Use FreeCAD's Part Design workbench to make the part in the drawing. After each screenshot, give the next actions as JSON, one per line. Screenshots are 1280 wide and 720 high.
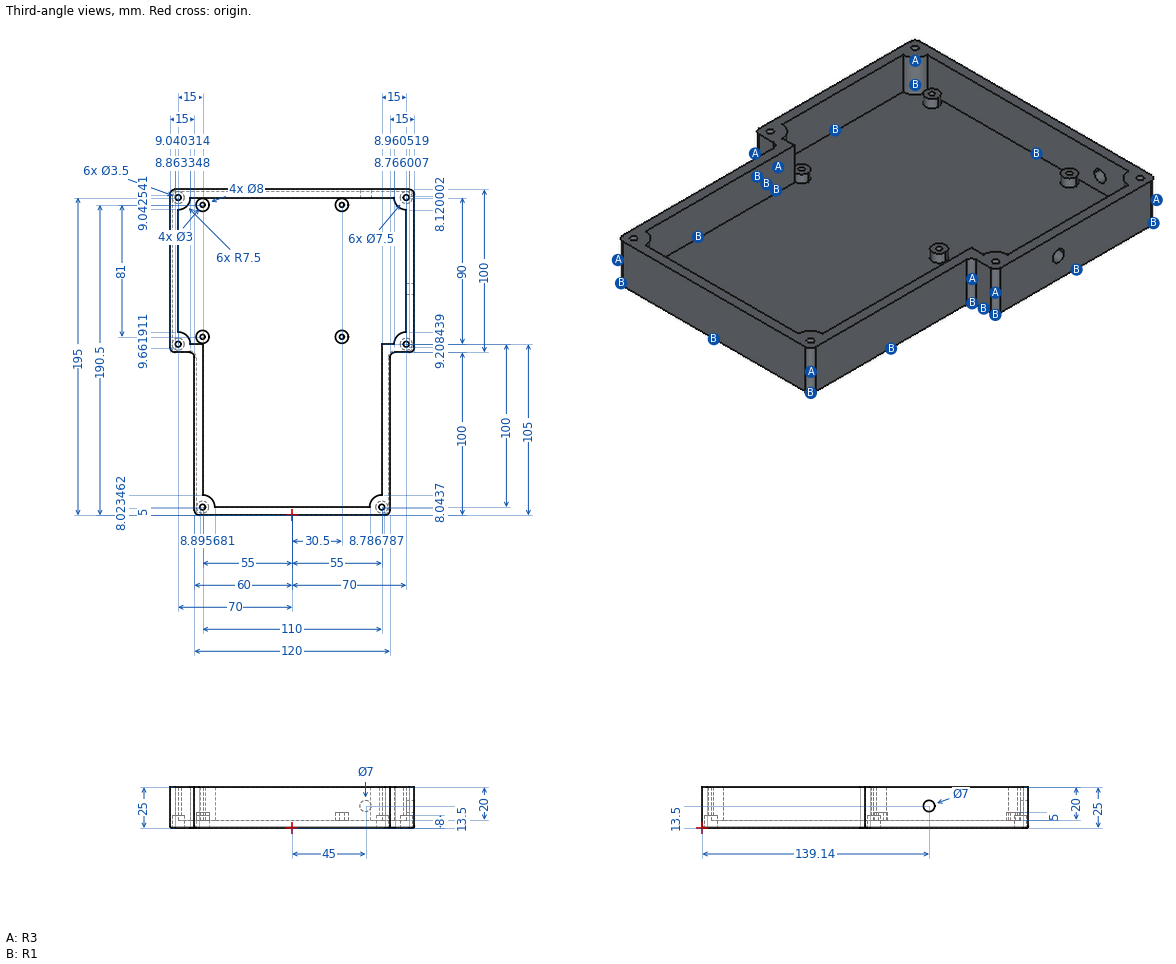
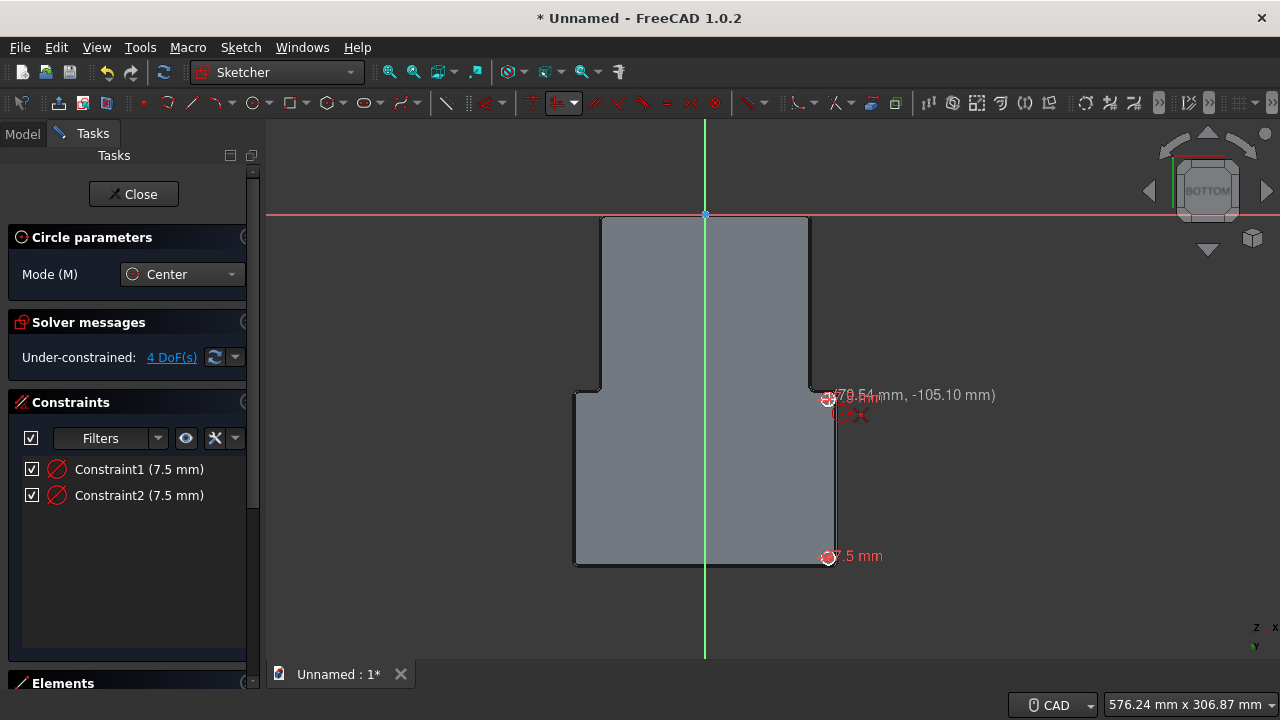
{"action": "scroll", "coordinate": [802, 223], "scroll_direction": "up", "scroll_amount": 7}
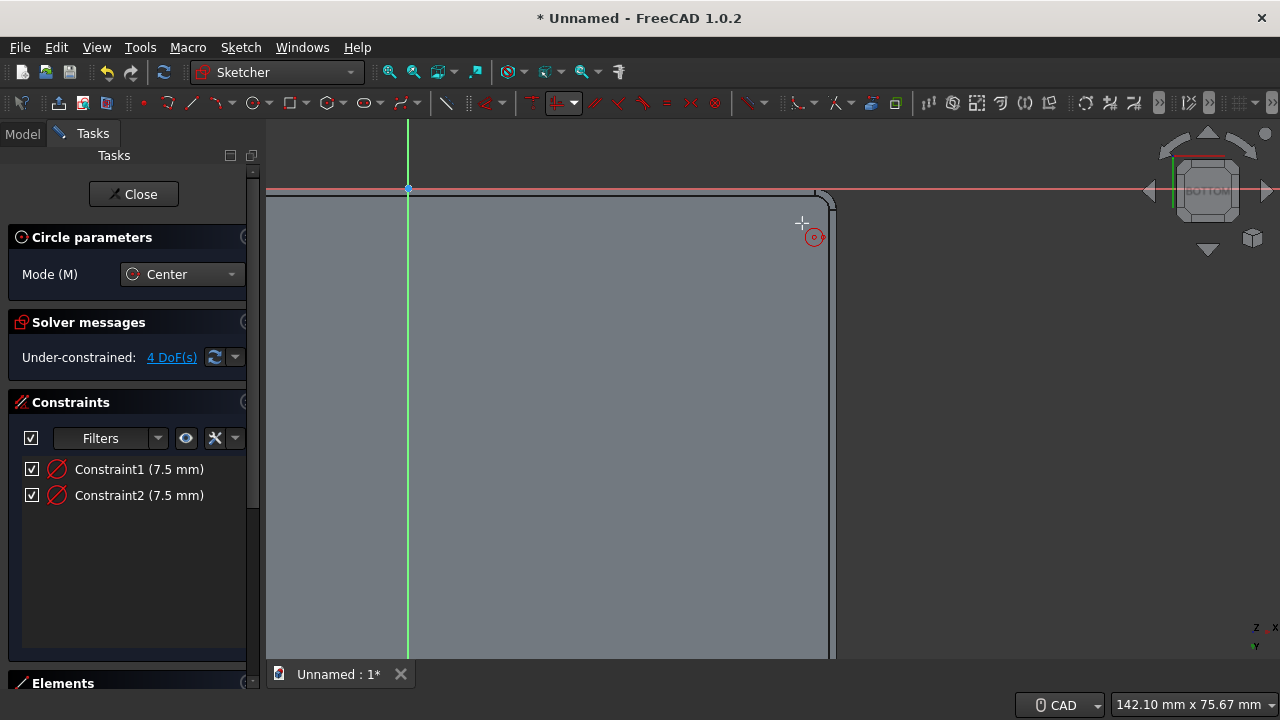
{"action": "left_click", "coordinate": [801, 224]}
{"action": "mouse_move", "coordinate": [820, 205]}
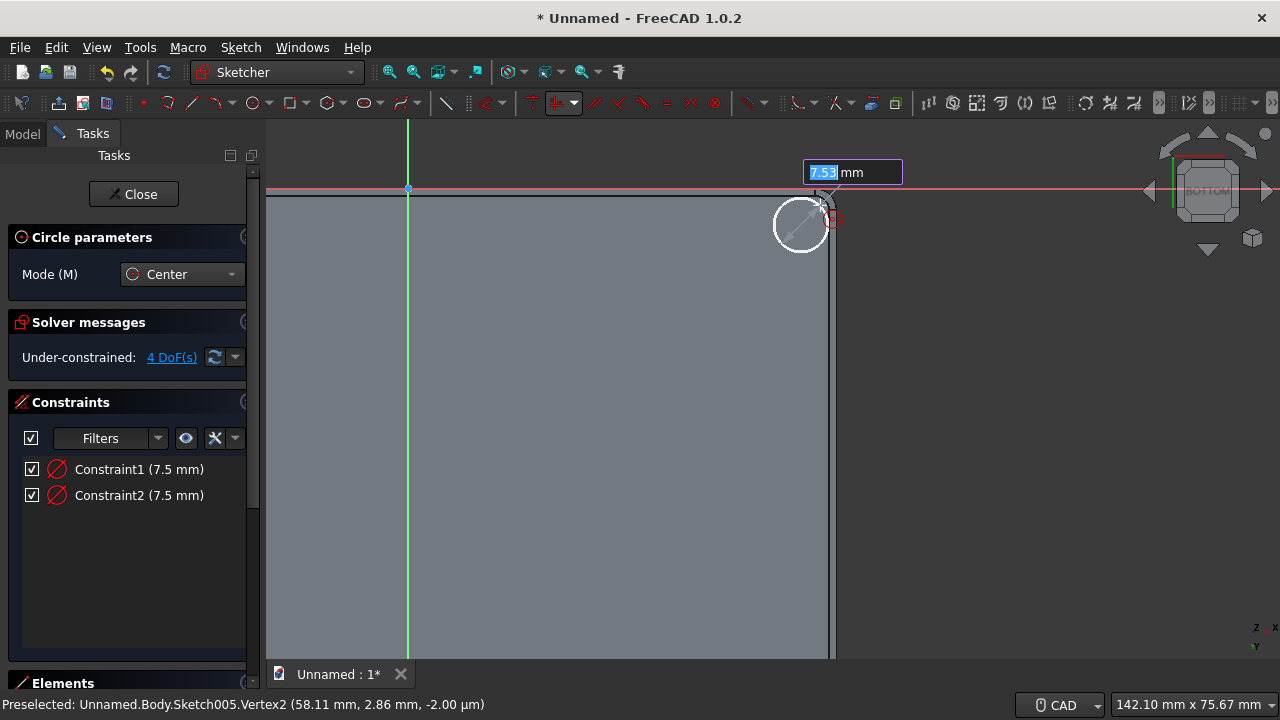
{"action": "type", "text": "7.5"}
{"action": "key", "text": "Return"}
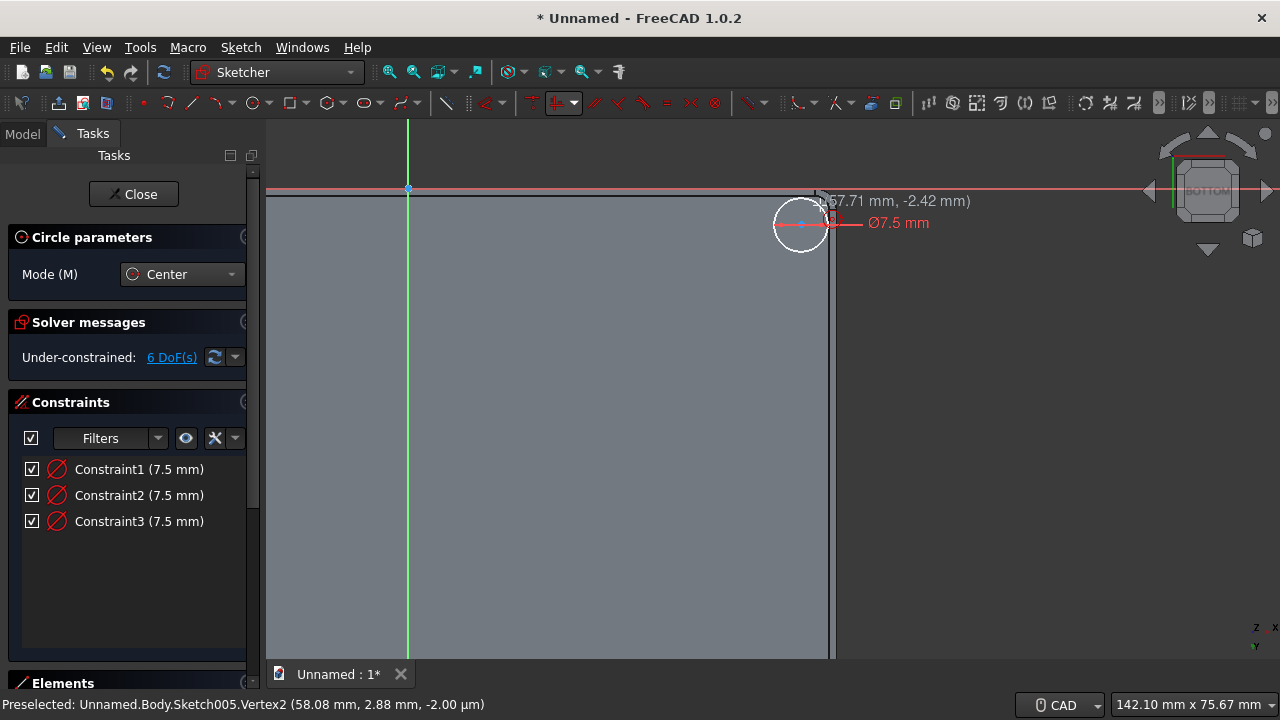
{"action": "scroll", "coordinate": [801, 222], "scroll_direction": "down", "scroll_amount": 7}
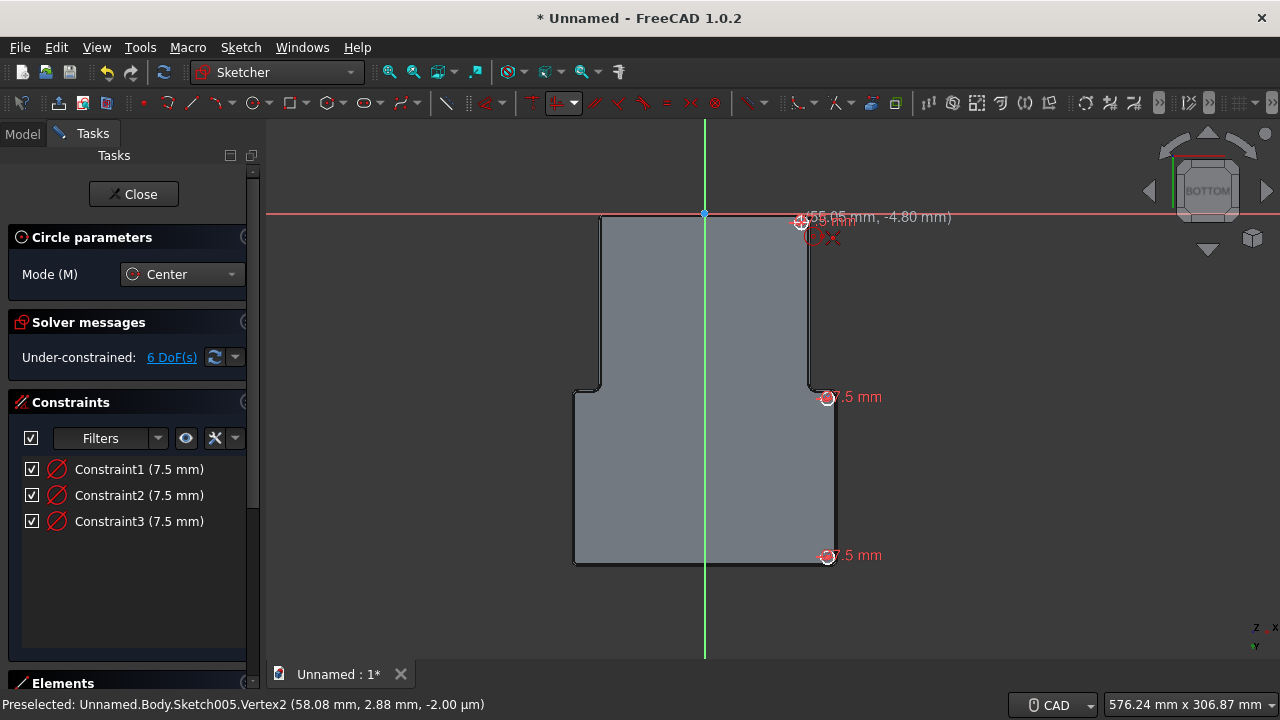
{"action": "scroll", "coordinate": [608, 223], "scroll_direction": "up", "scroll_amount": 7}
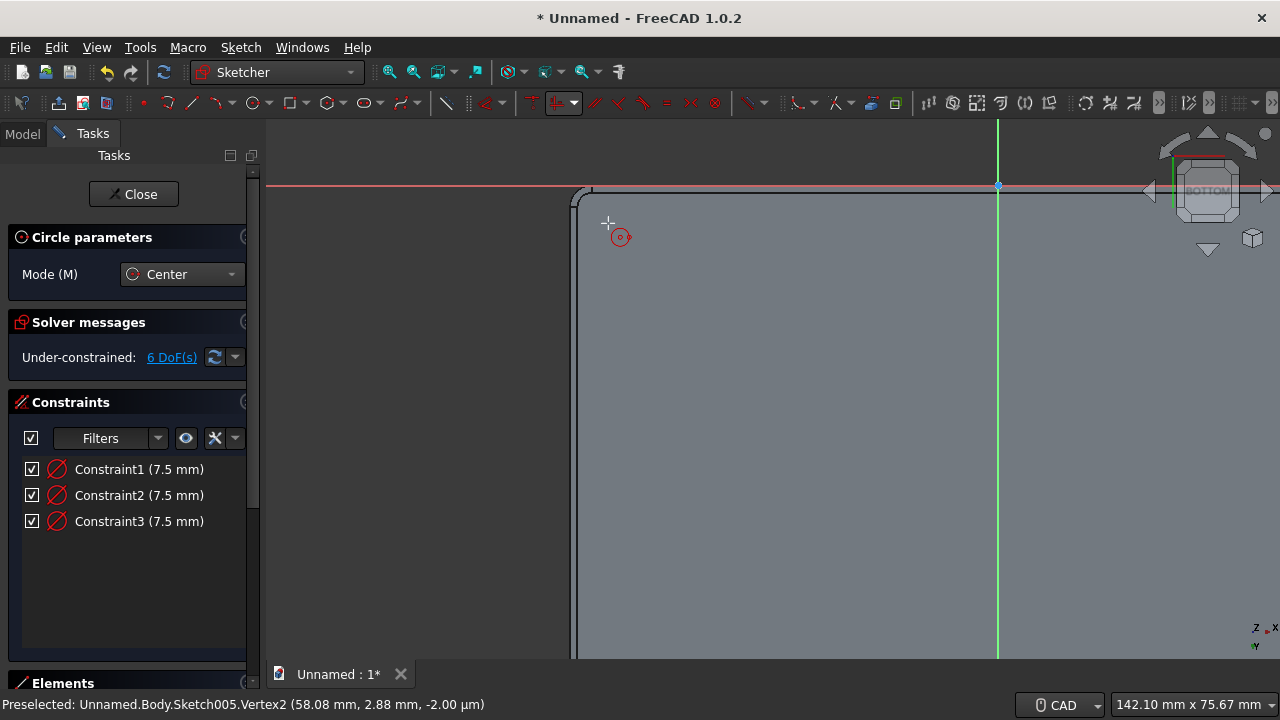
{"action": "left_click", "coordinate": [606, 221]}
{"action": "mouse_move", "coordinate": [625, 202]}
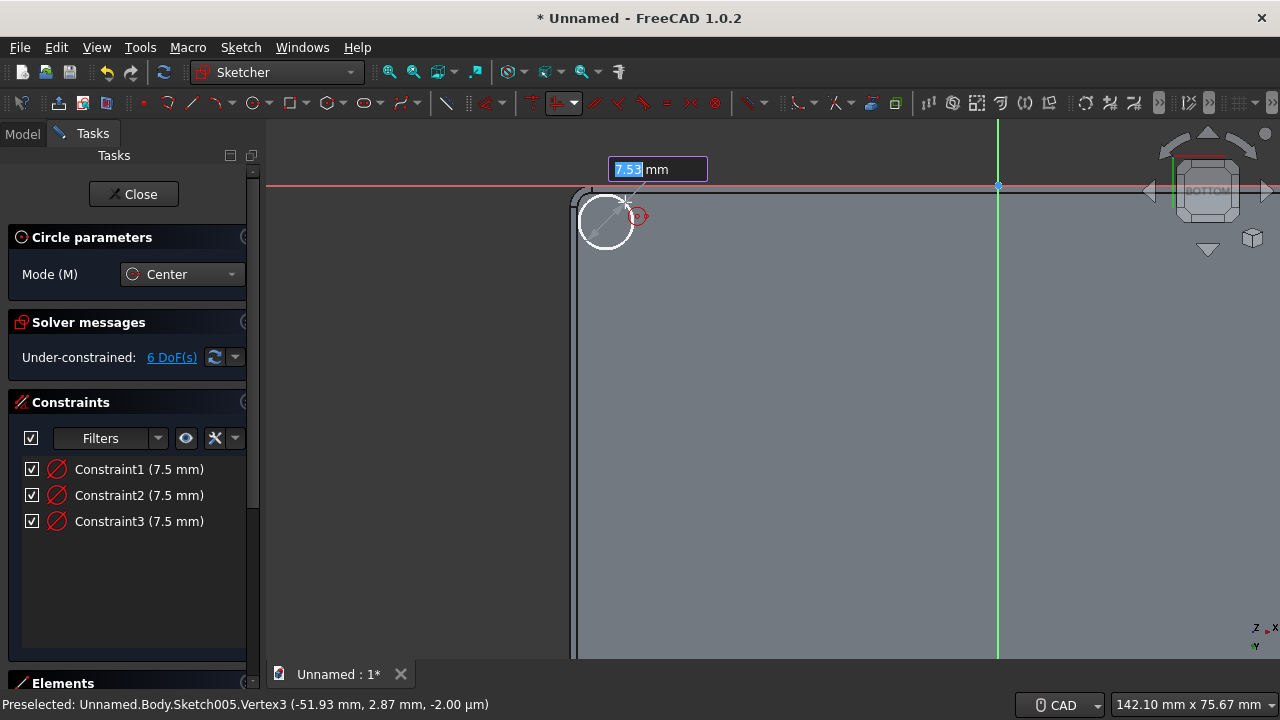
{"action": "type", "text": "7.5"}
{"action": "key", "text": "Return"}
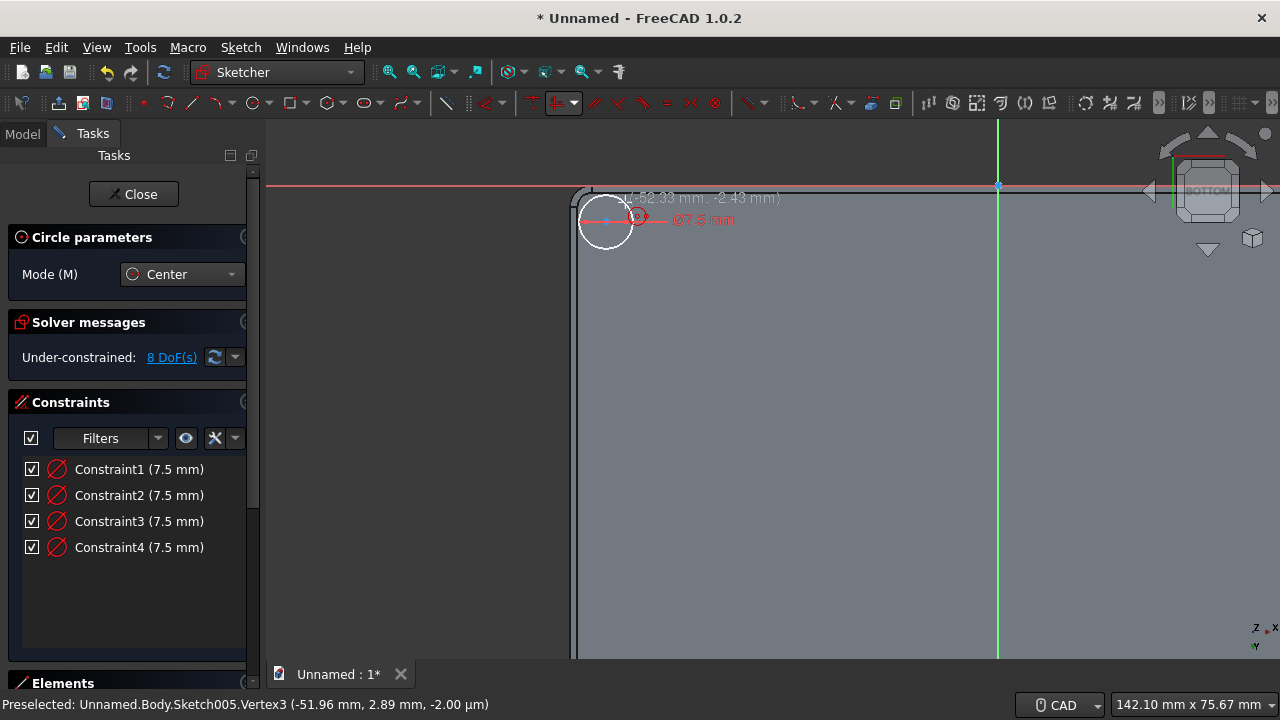
{"action": "scroll", "coordinate": [608, 223], "scroll_direction": "down", "scroll_amount": 7}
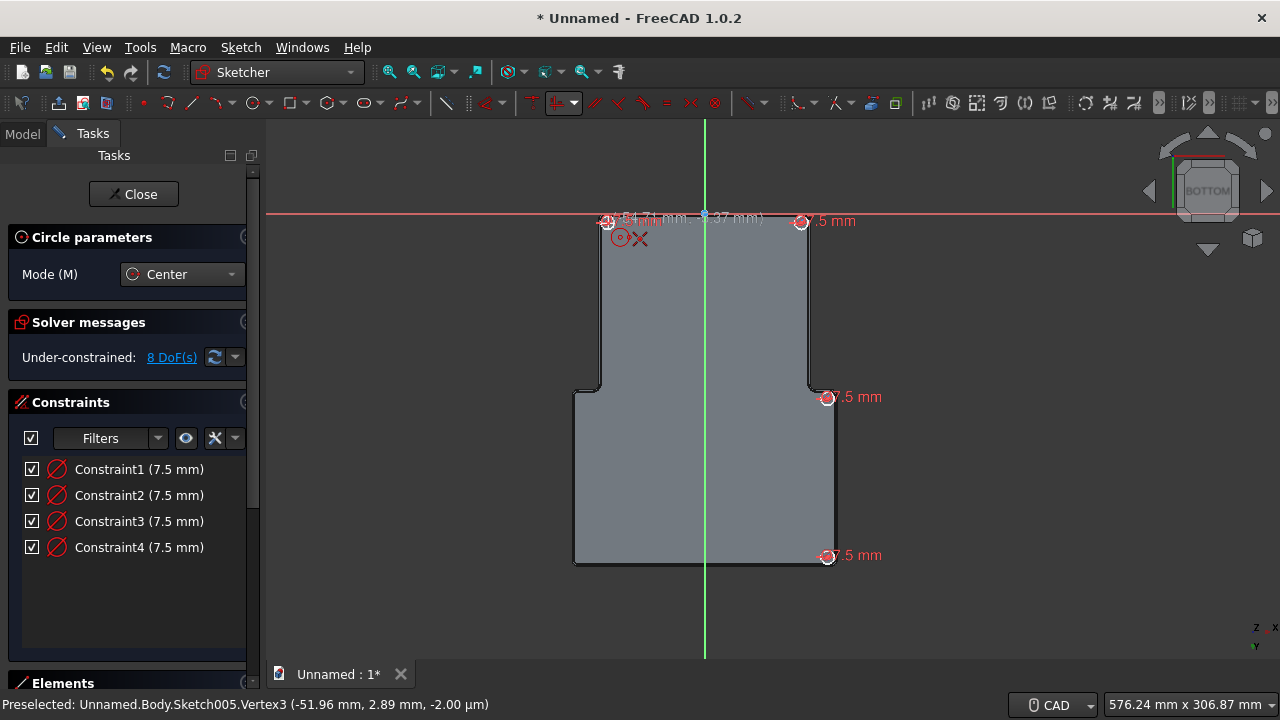
{"action": "scroll", "coordinate": [581, 399], "scroll_direction": "up", "scroll_amount": 7}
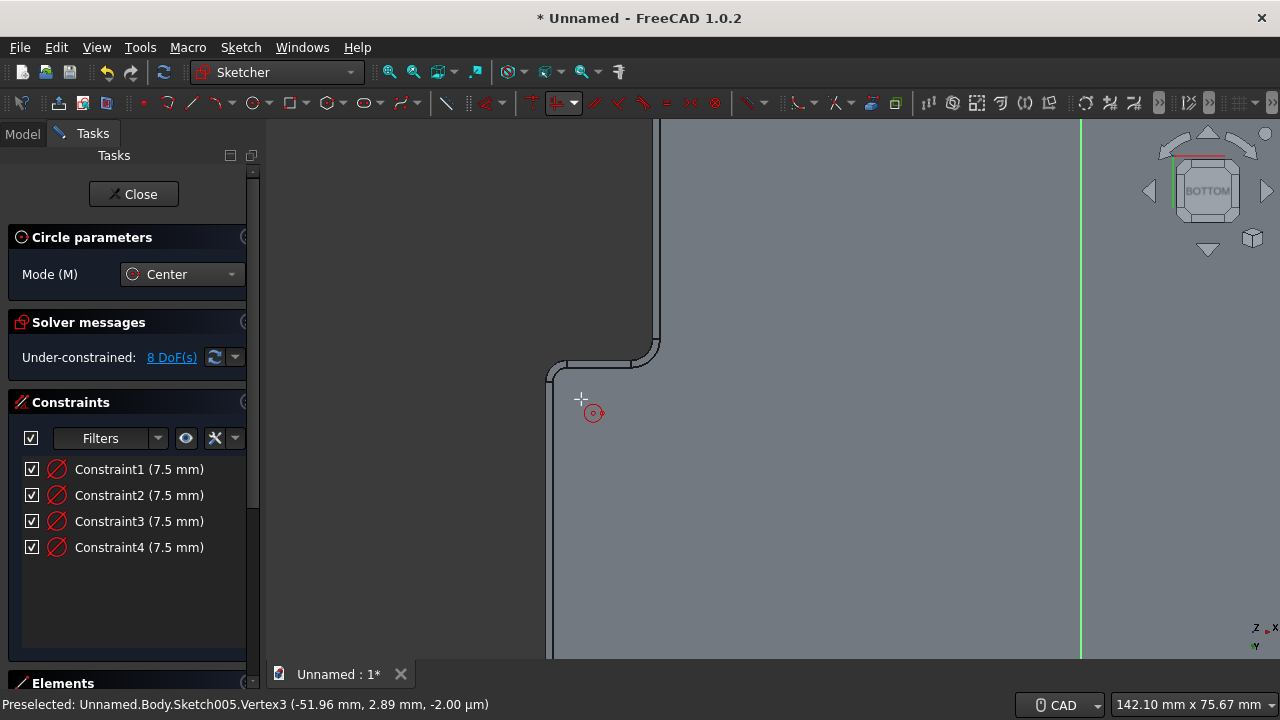
{"action": "left_click", "coordinate": [581, 396]}
{"action": "mouse_move", "coordinate": [600, 377]}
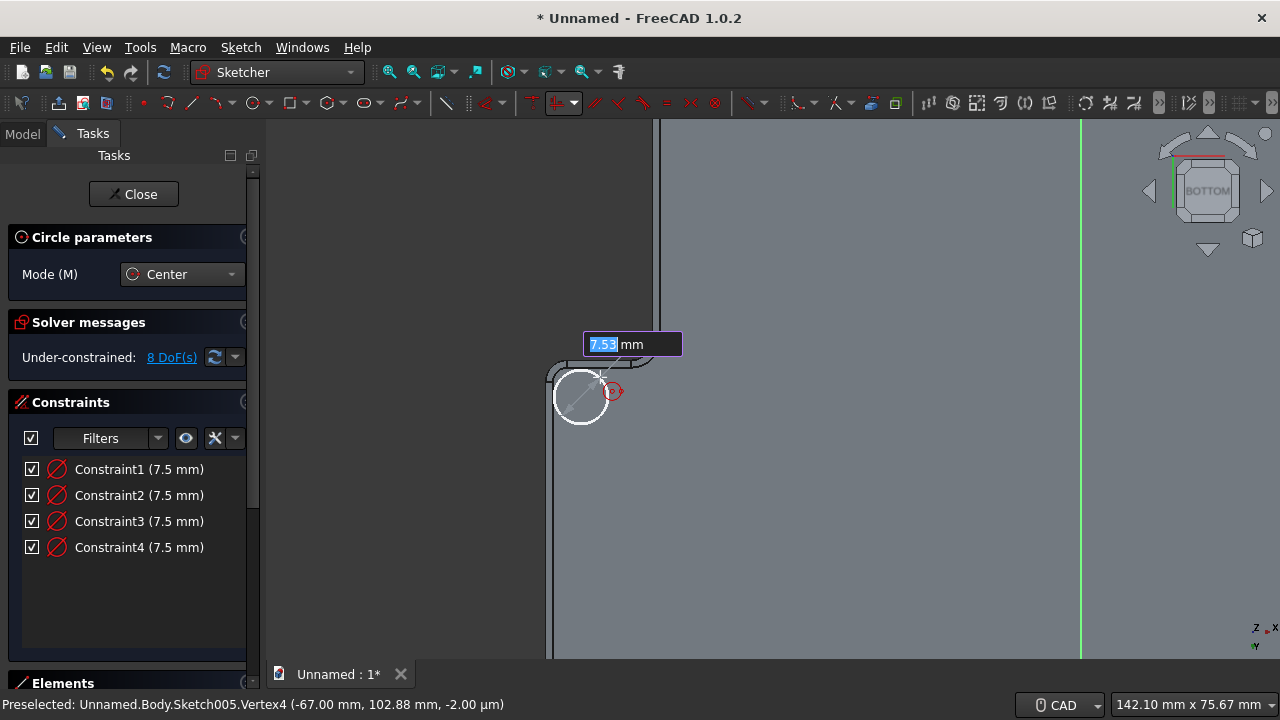
{"action": "type", "text": "7.5"}
{"action": "key", "text": "Return"}